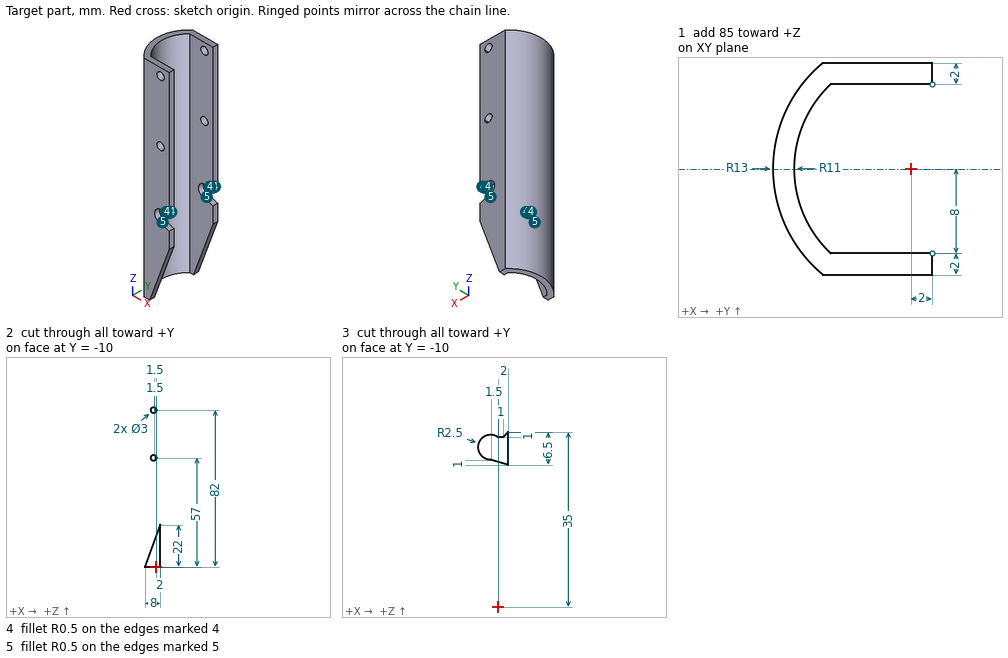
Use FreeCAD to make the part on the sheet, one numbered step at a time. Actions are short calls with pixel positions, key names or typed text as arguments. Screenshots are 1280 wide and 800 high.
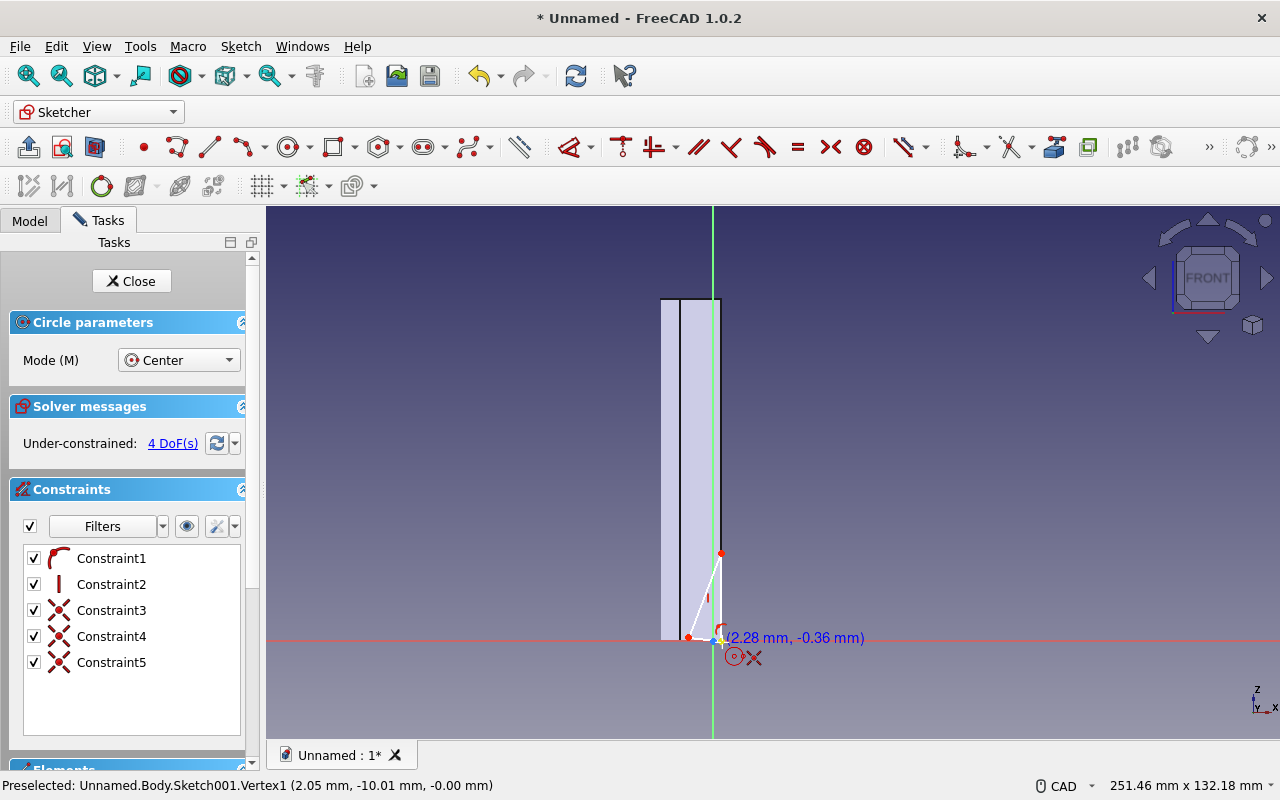
scroll(707, 311, up, 7)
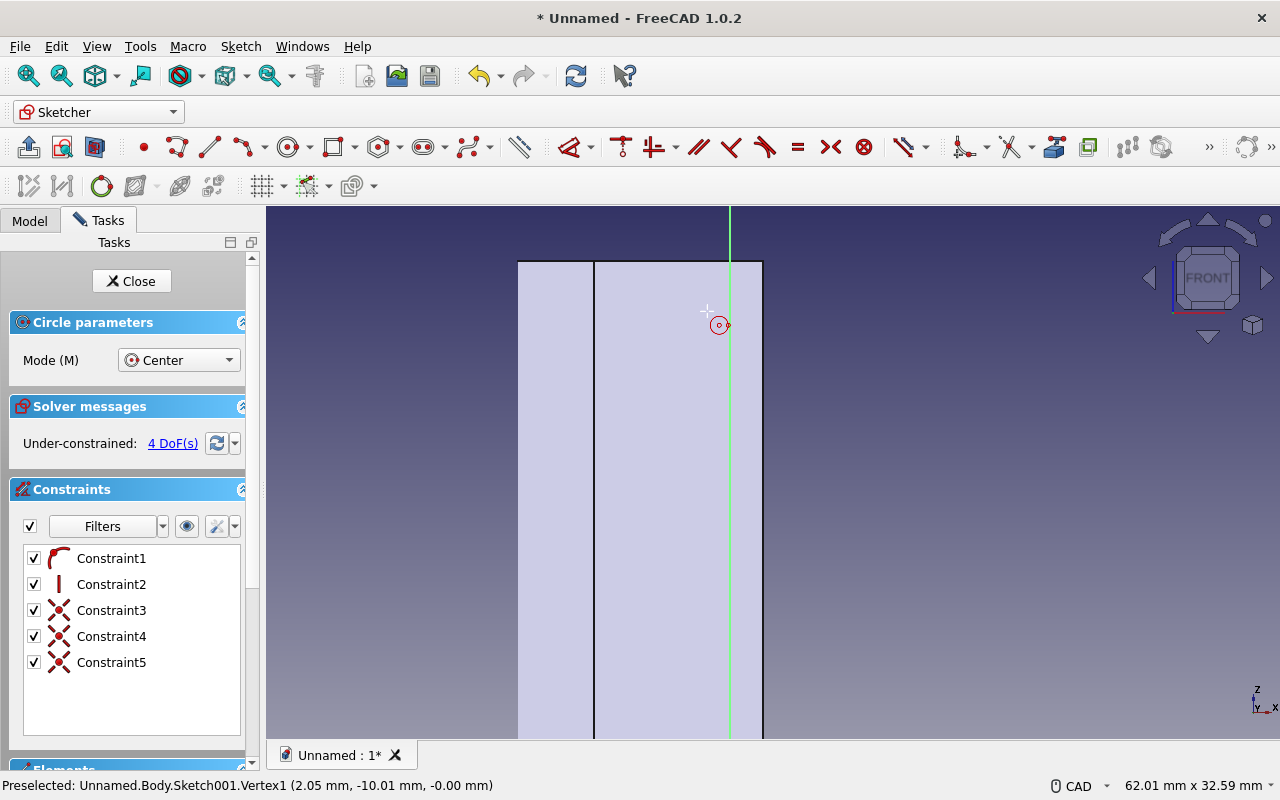
click(706, 310)
move(688, 292)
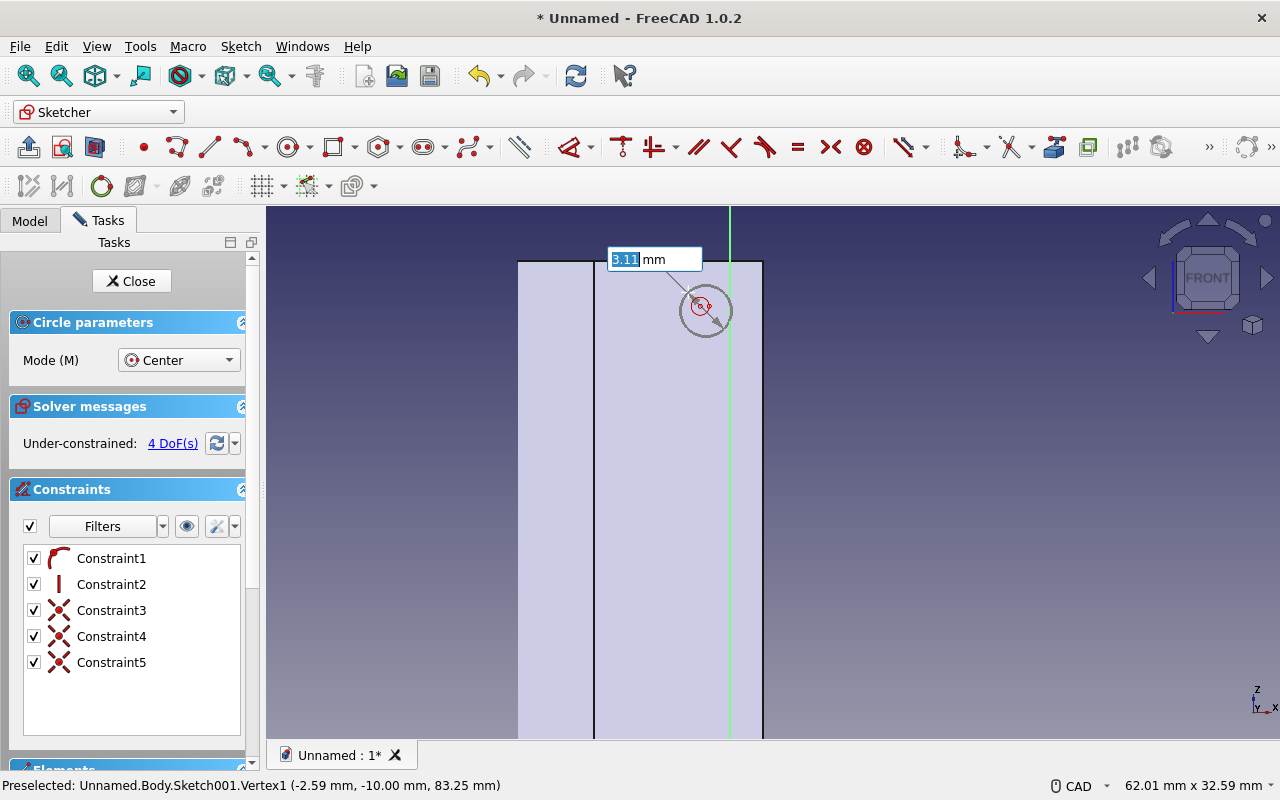
text(3)
key(Return)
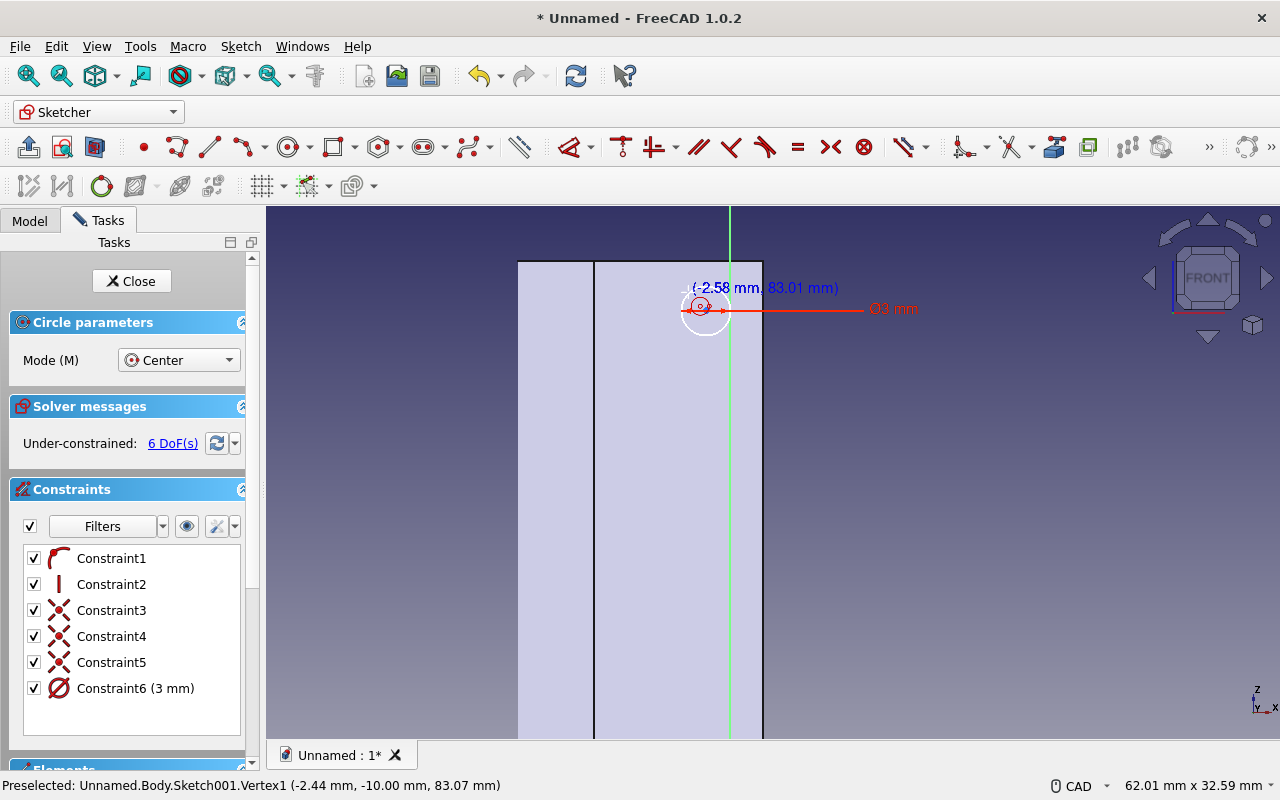
scroll(707, 310, down, 7)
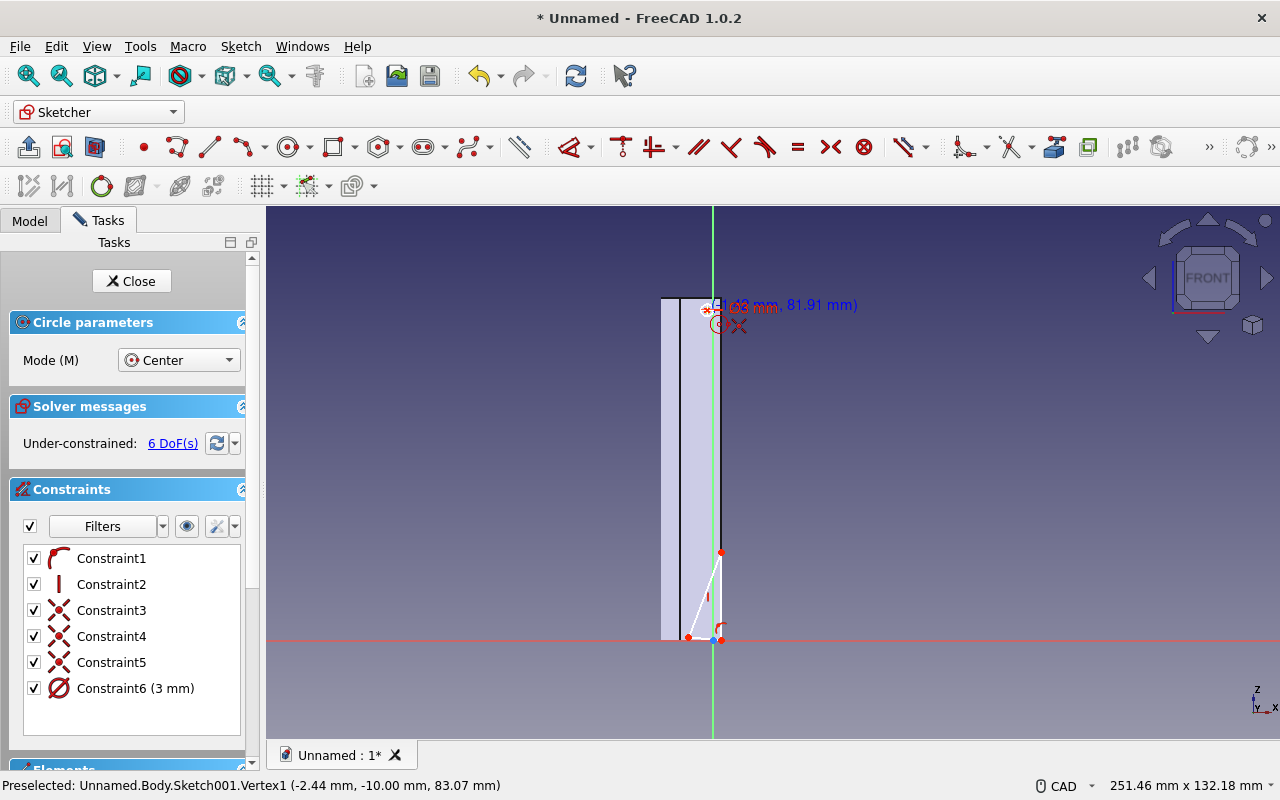
scroll(707, 411, up, 7)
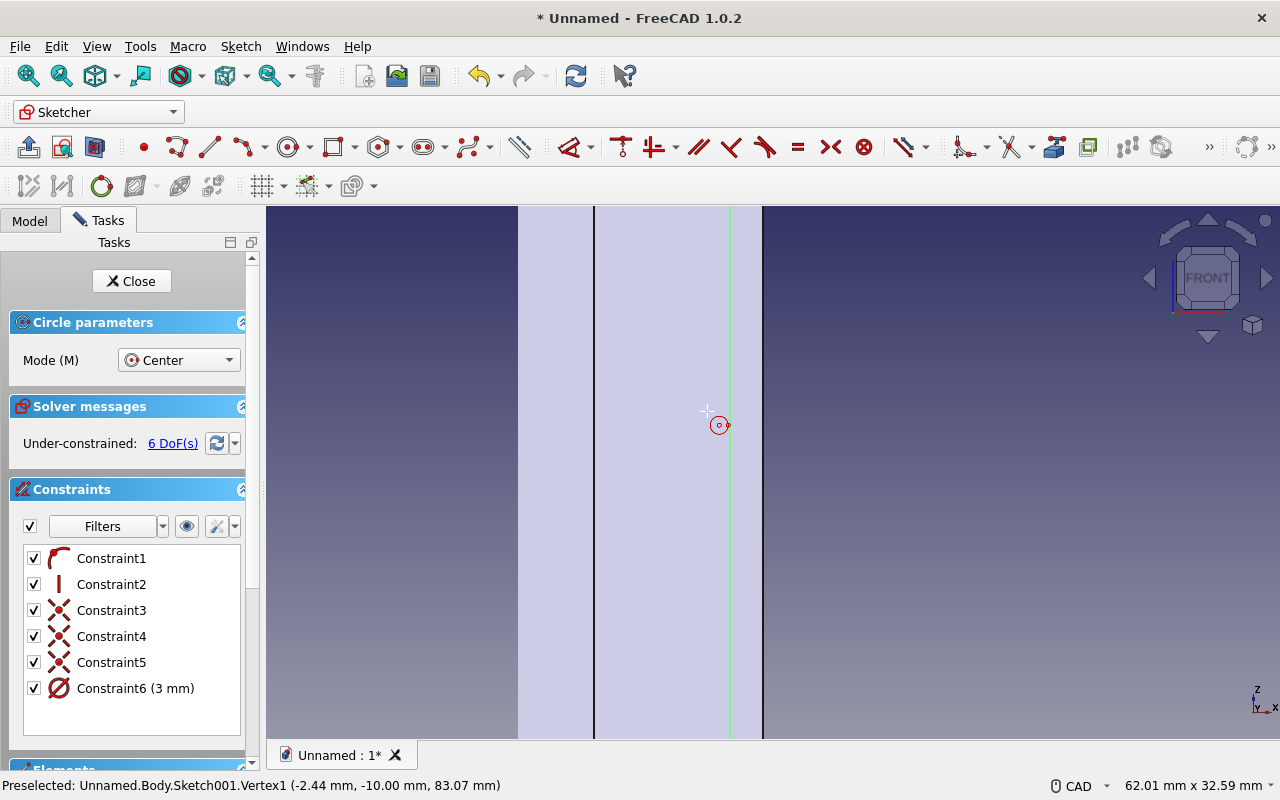
click(706, 409)
move(688, 392)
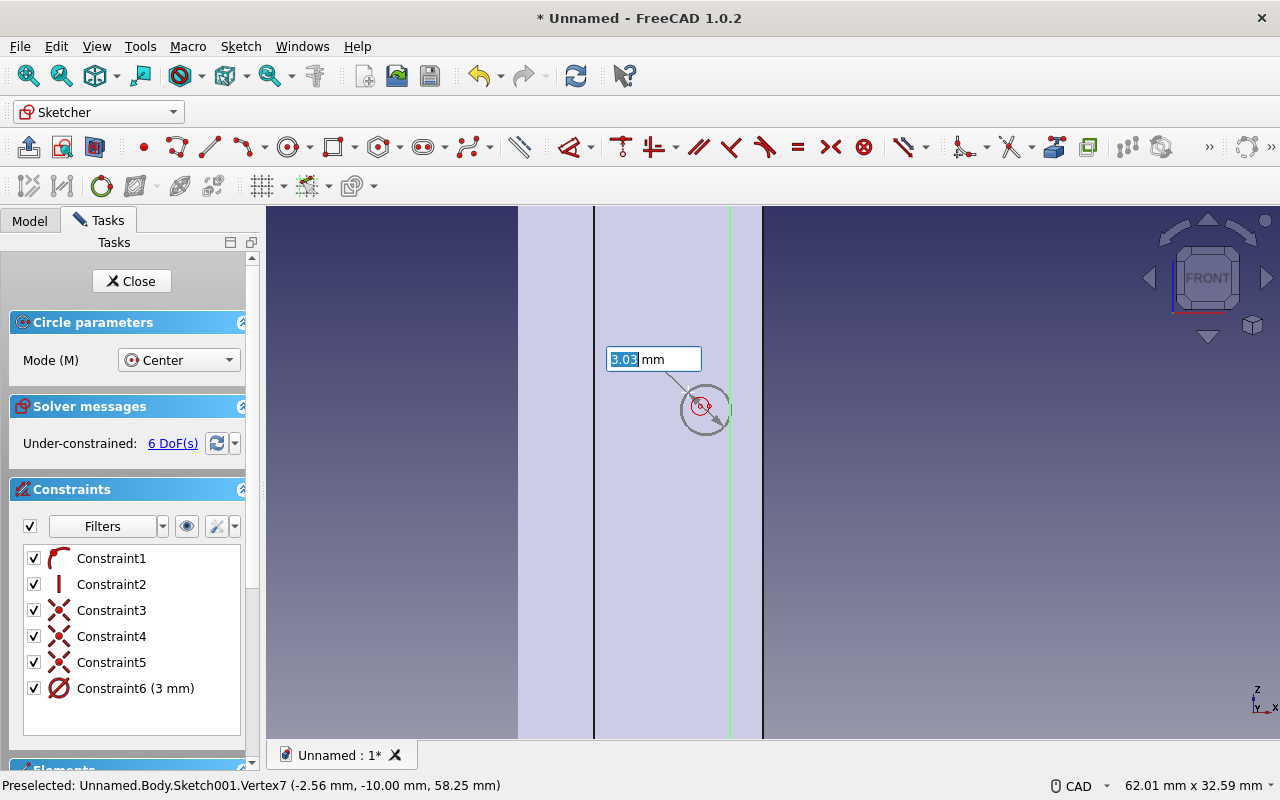
text(3)
key(Return)
key(Escape)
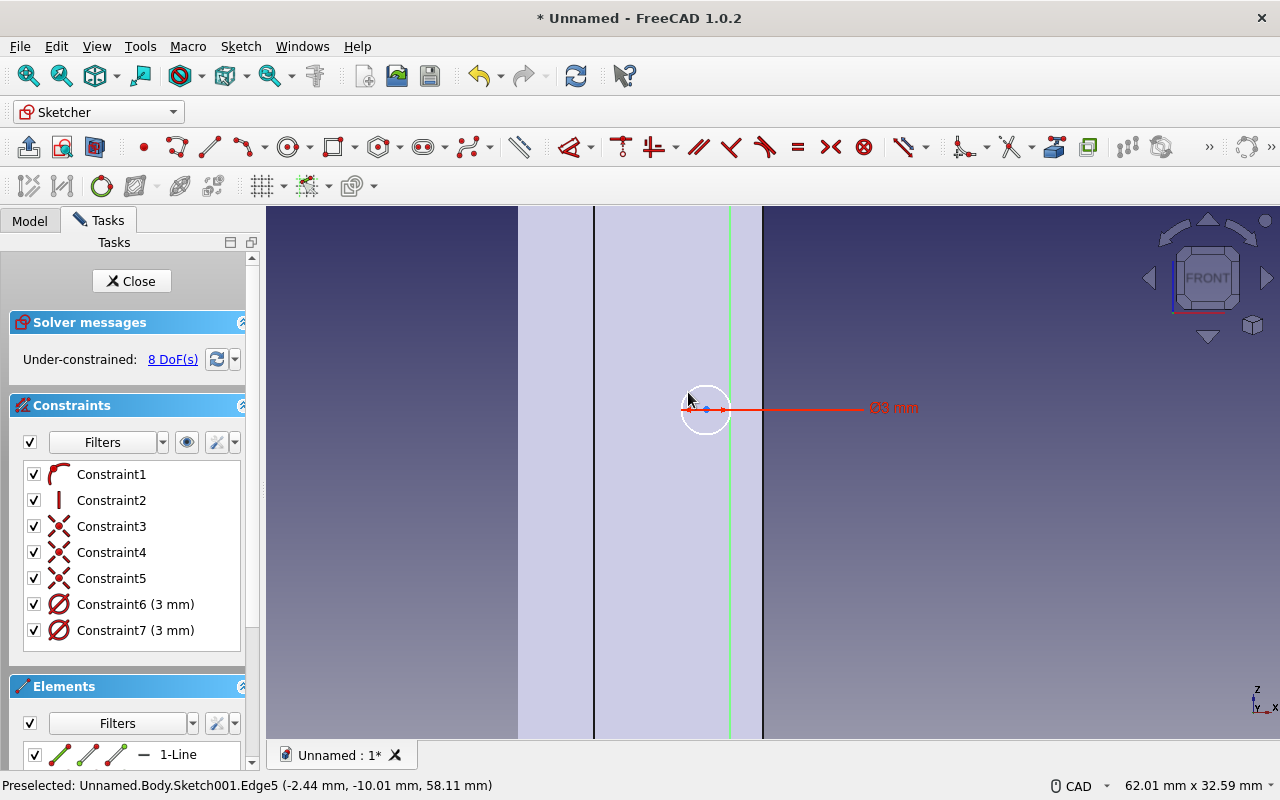
scroll(707, 412, down, 7)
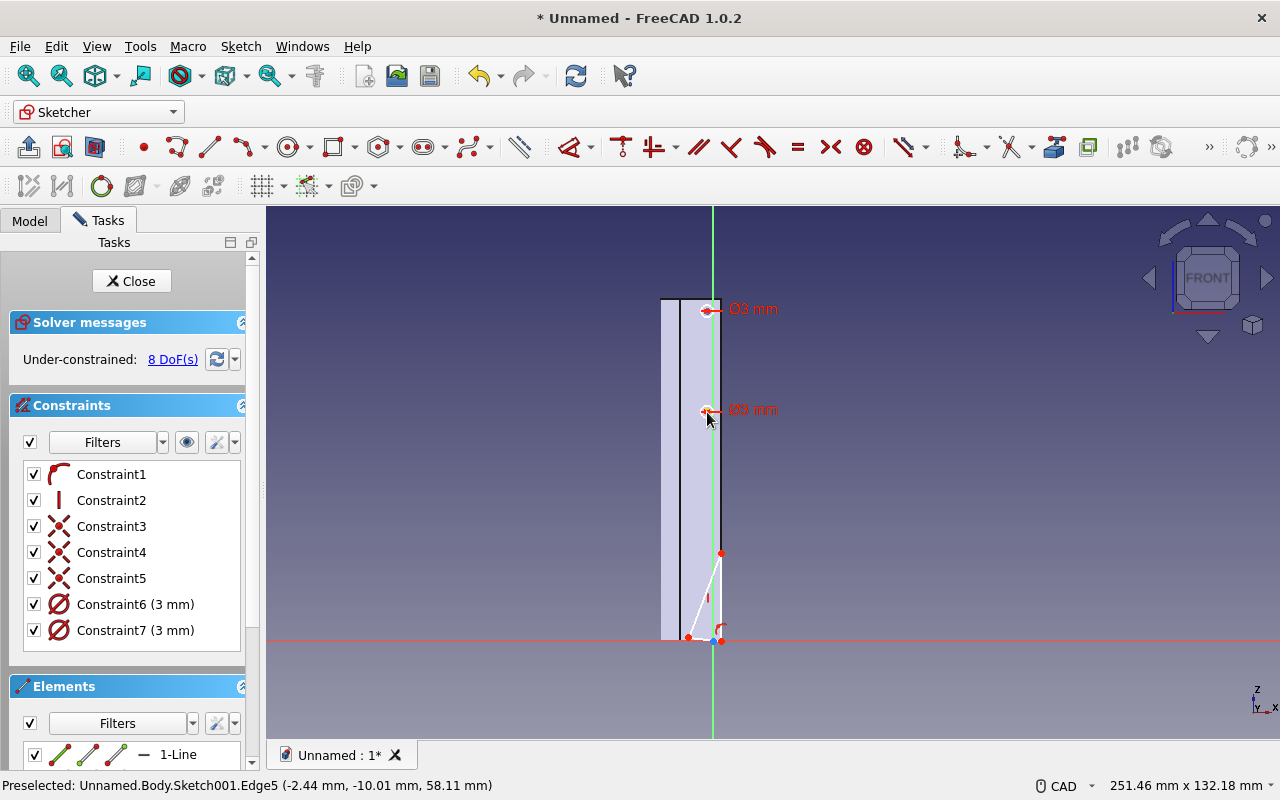
scroll(699, 639, up, 9)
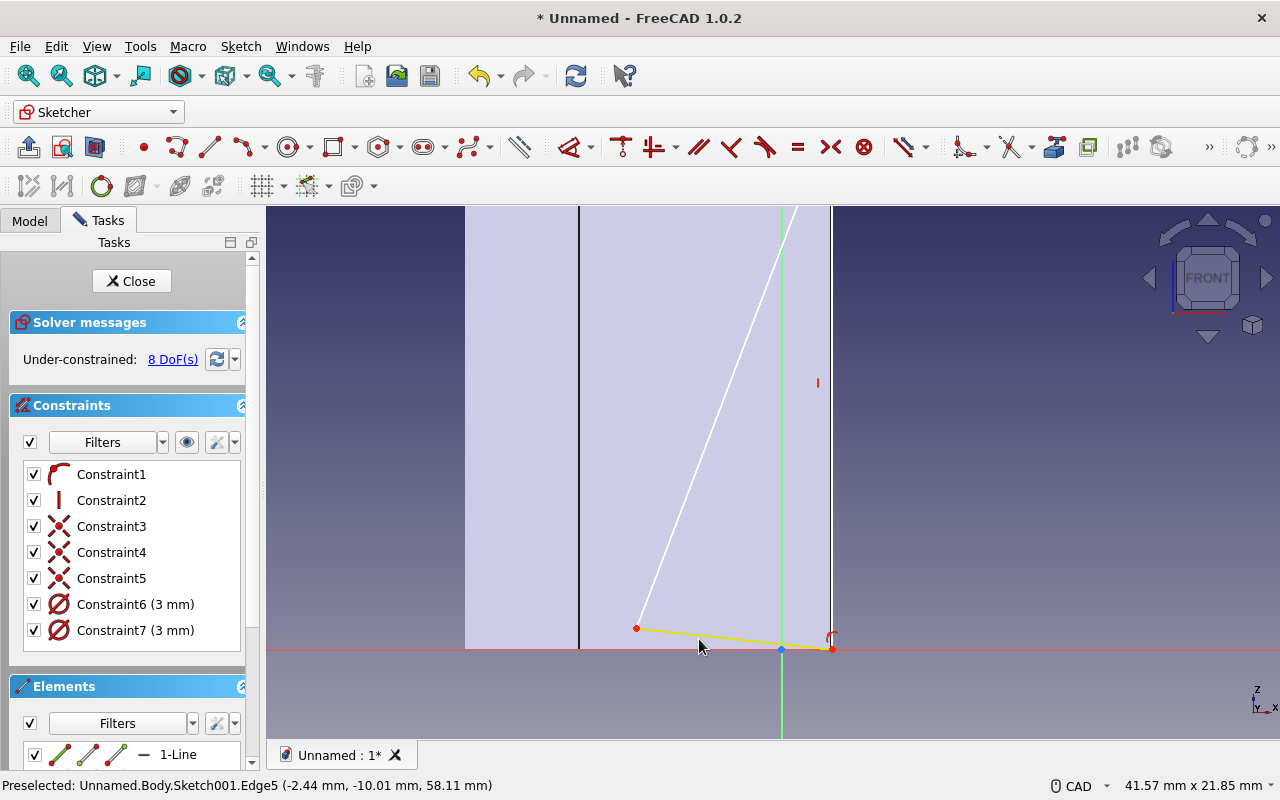
click(695, 635)